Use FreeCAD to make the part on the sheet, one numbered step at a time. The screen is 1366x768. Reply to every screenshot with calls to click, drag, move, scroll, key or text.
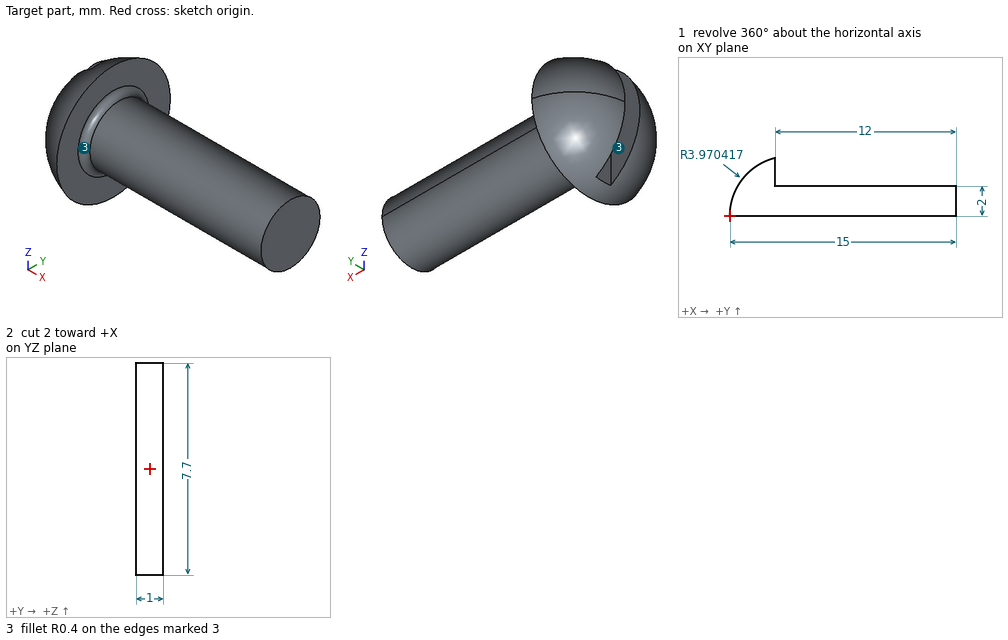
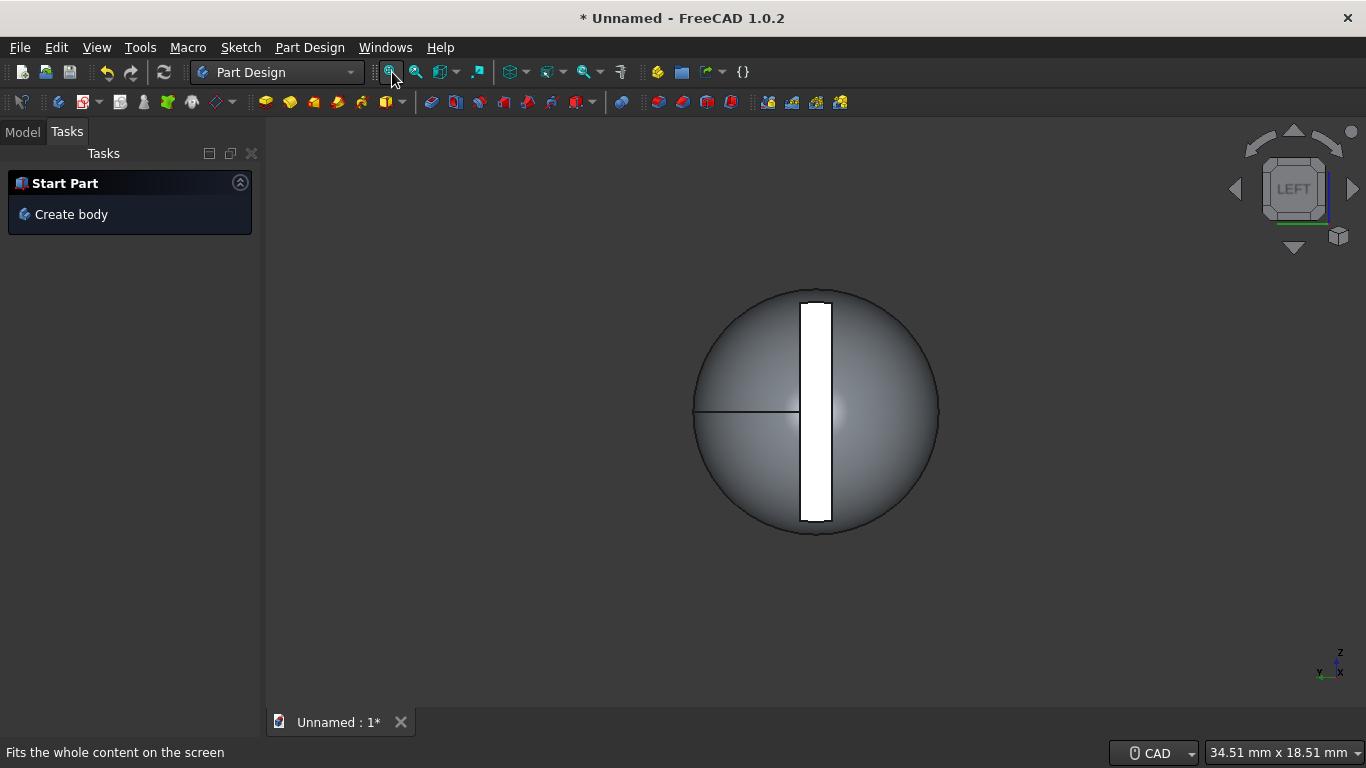
key(0)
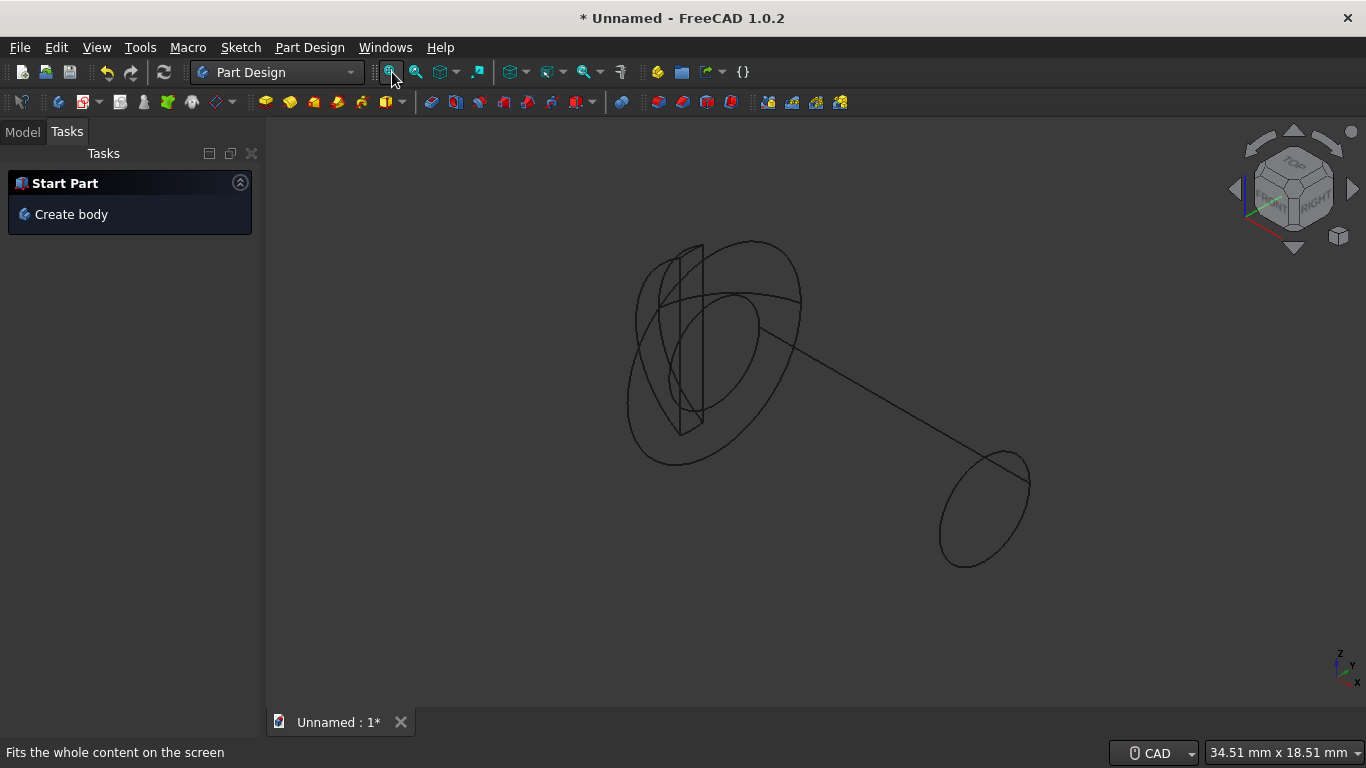
click(669, 378)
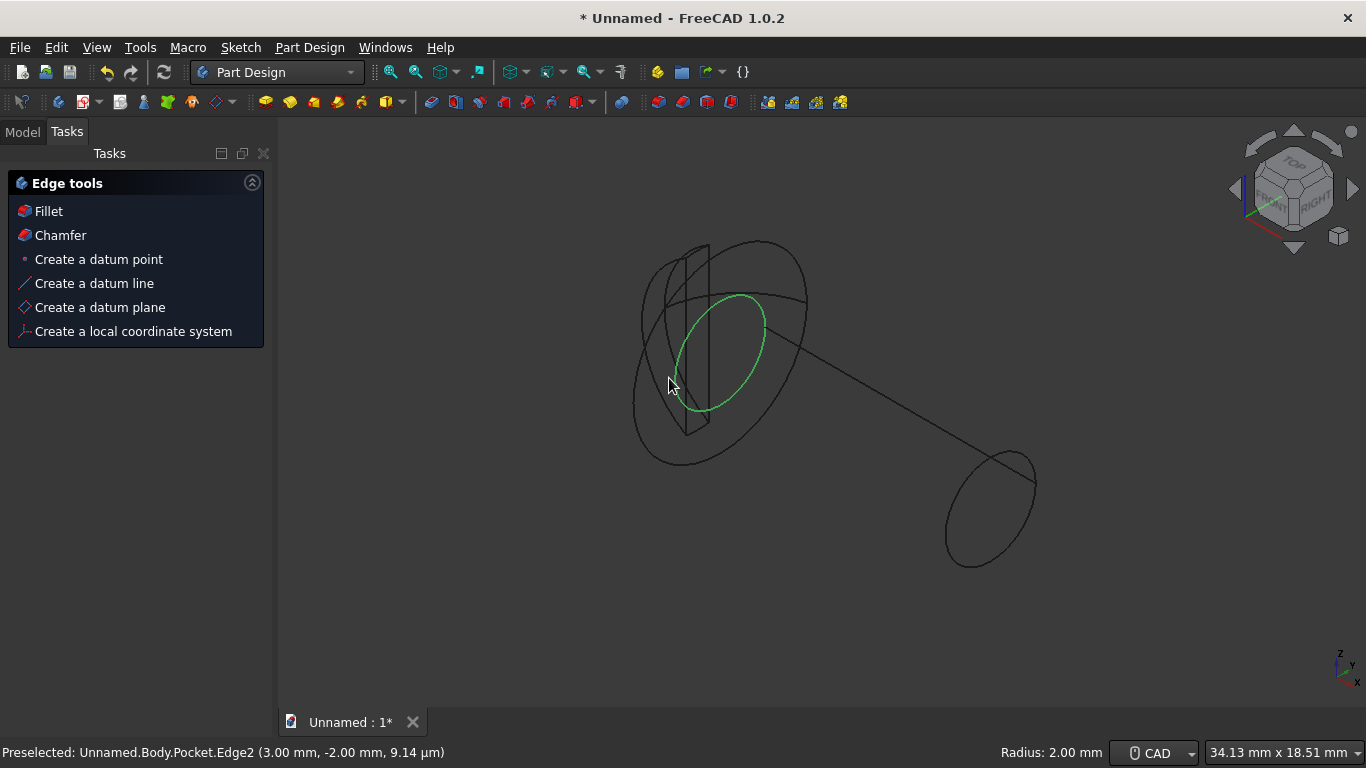
key(v)
key(1)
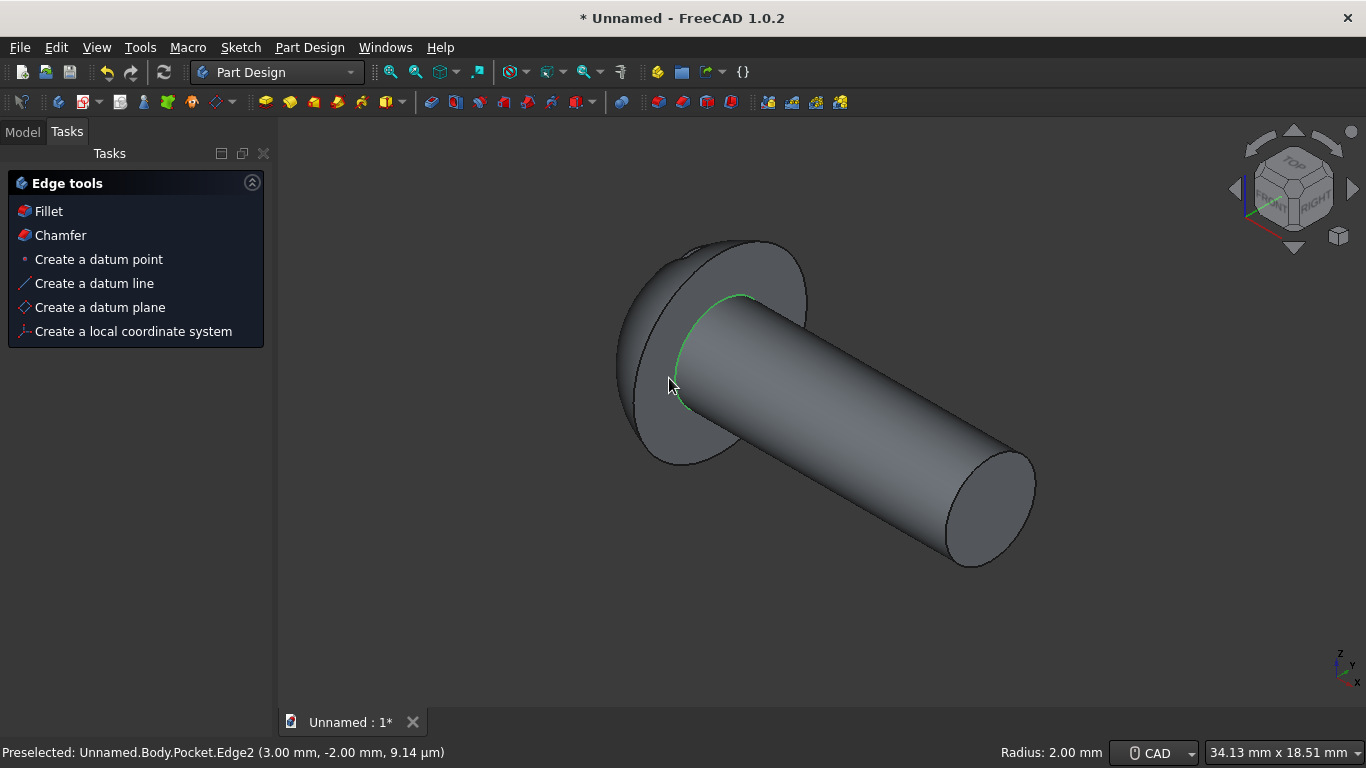
click(660, 102)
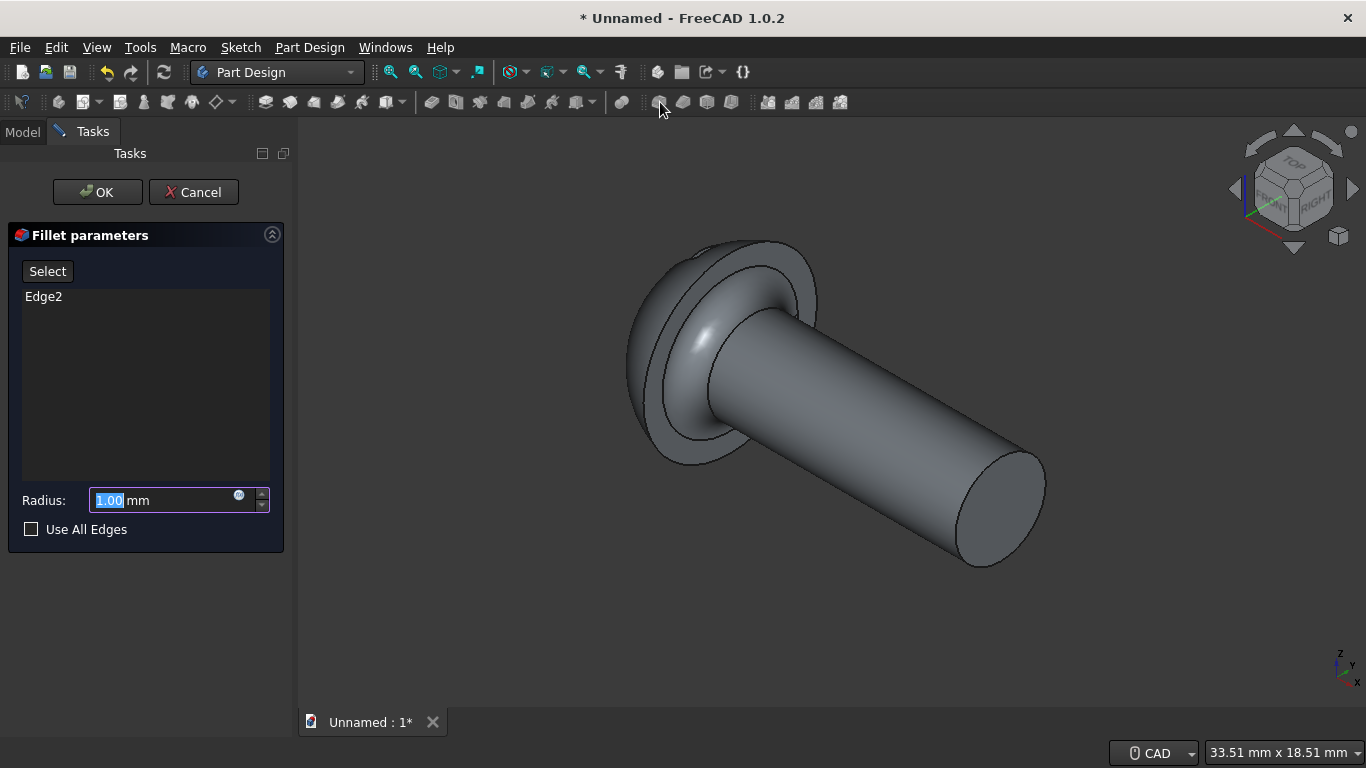
text(0.4)
key(Tab)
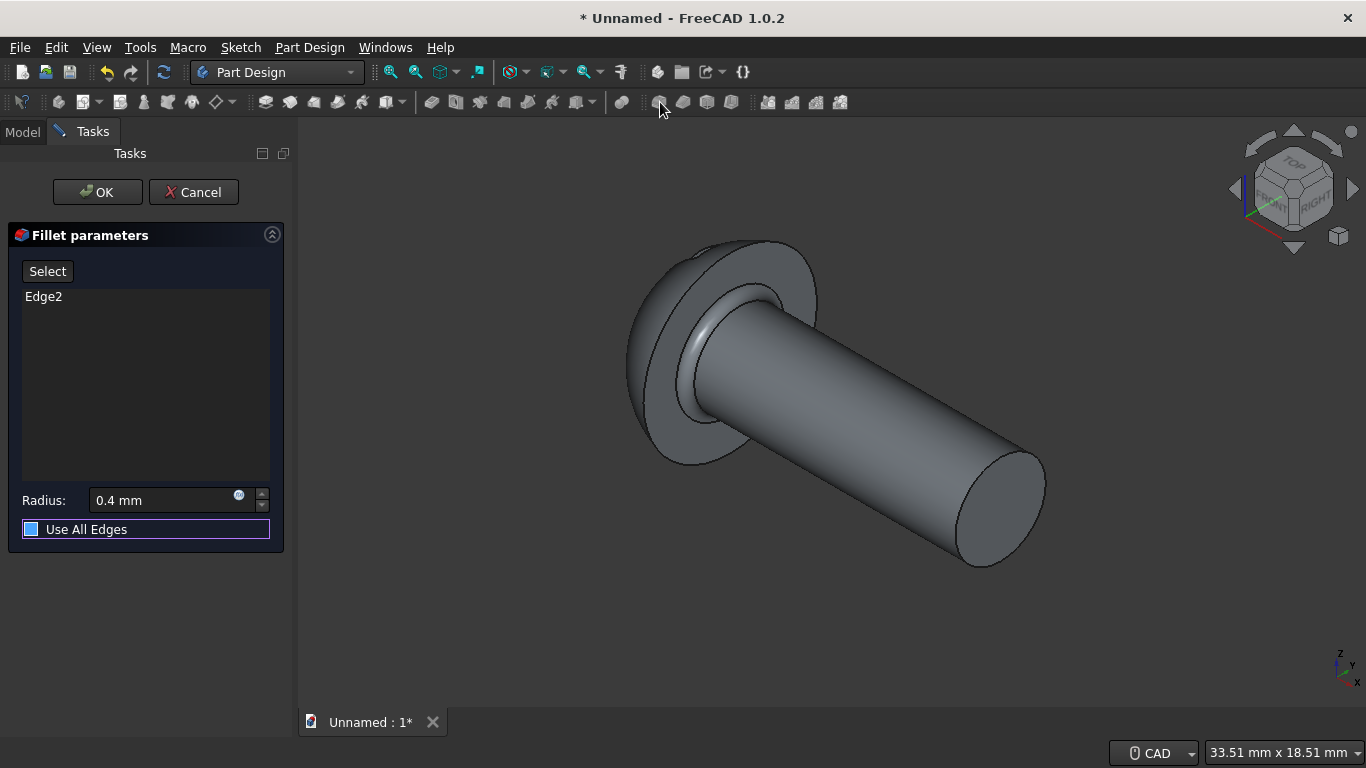
click(98, 192)